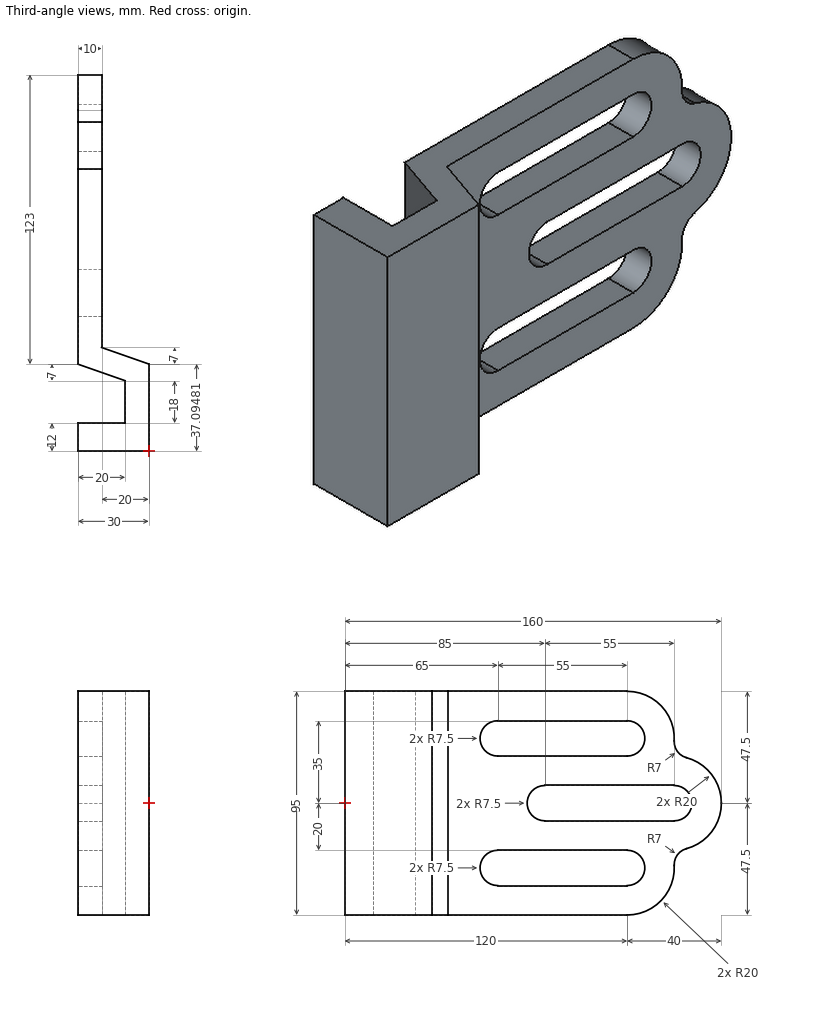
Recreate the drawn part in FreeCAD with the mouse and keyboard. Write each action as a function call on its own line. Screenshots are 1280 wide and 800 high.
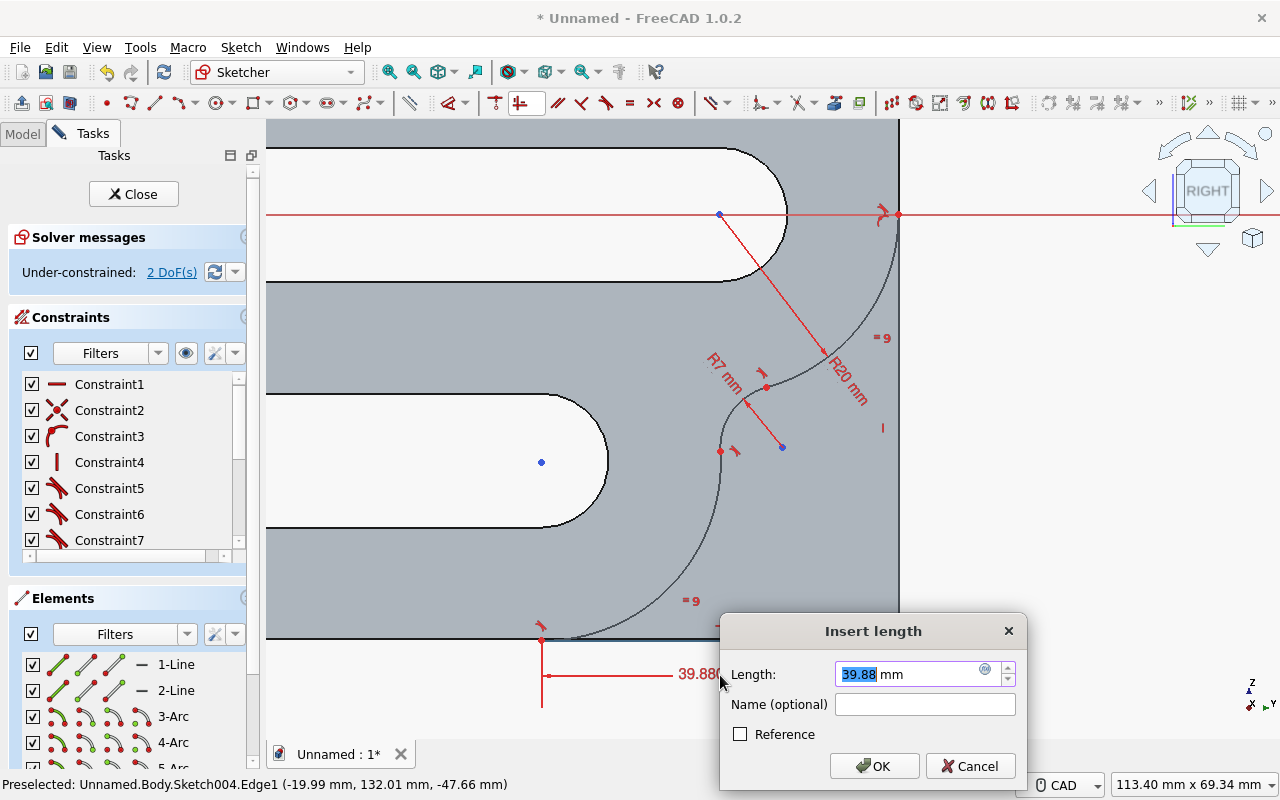
text(40)
key(Return)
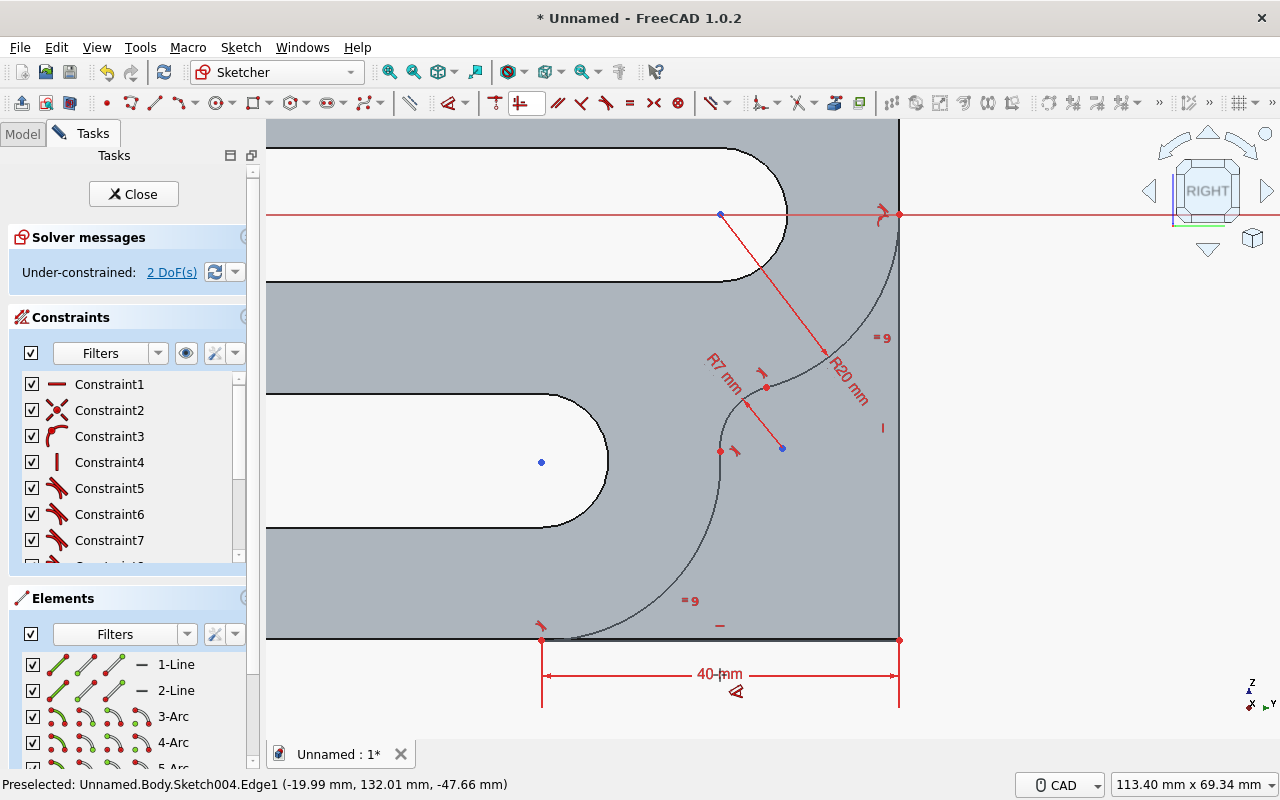
click(899, 513)
click(933, 428)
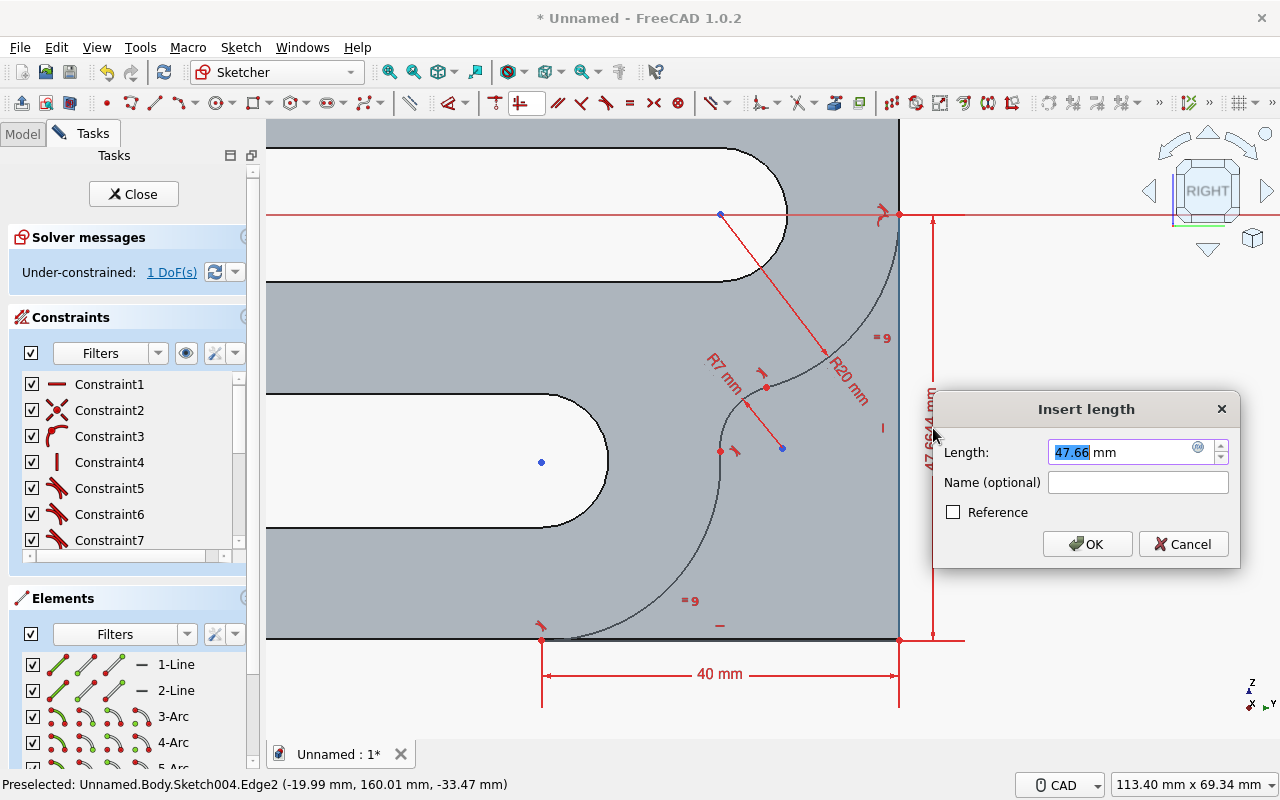
text(47.5)
key(Return)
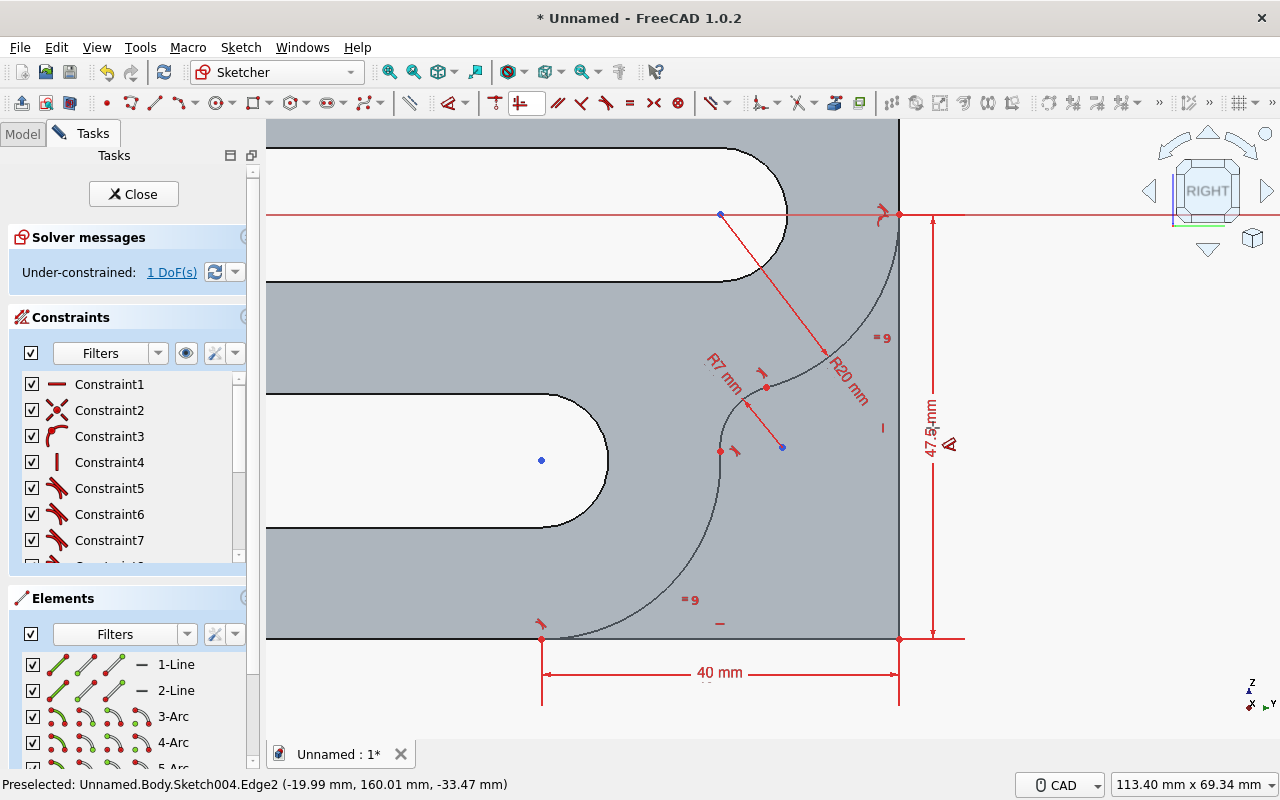
click(542, 639)
click(418, 673)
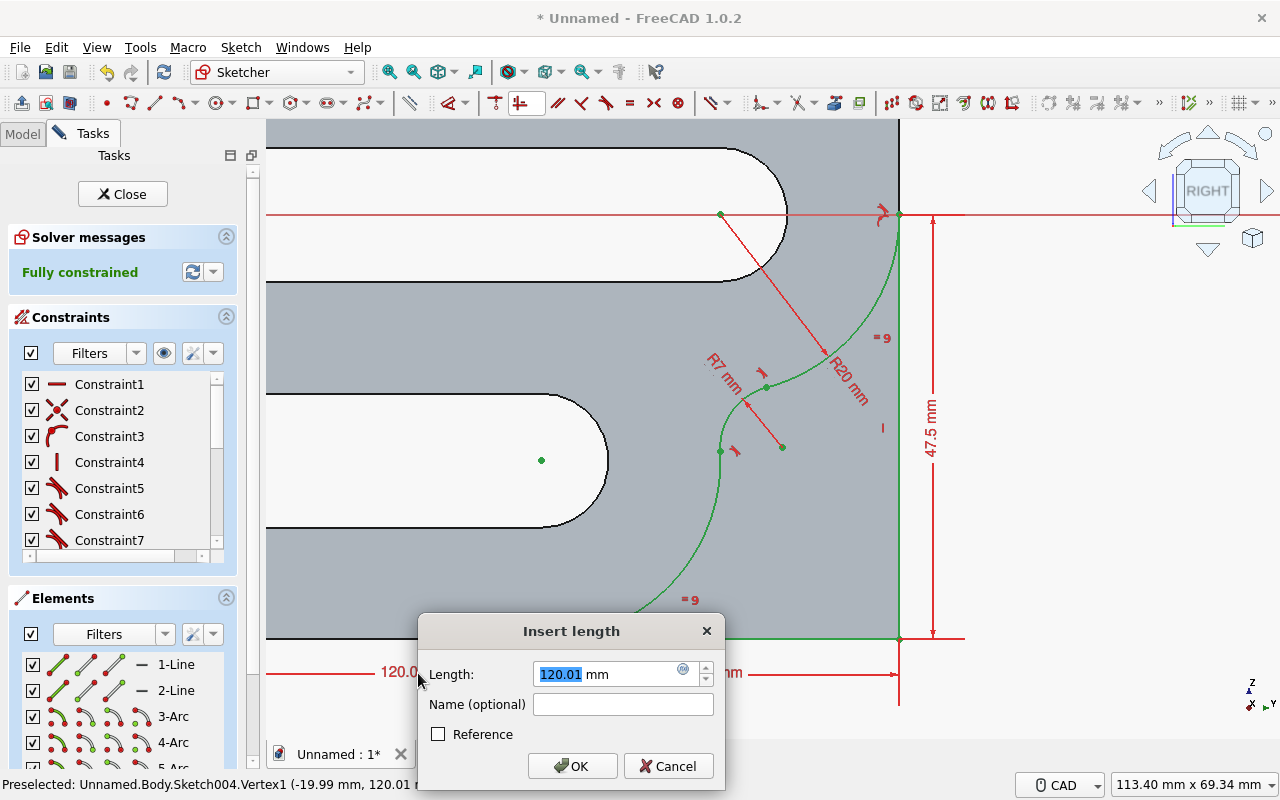
text(120)
key(Return)
key(Escape)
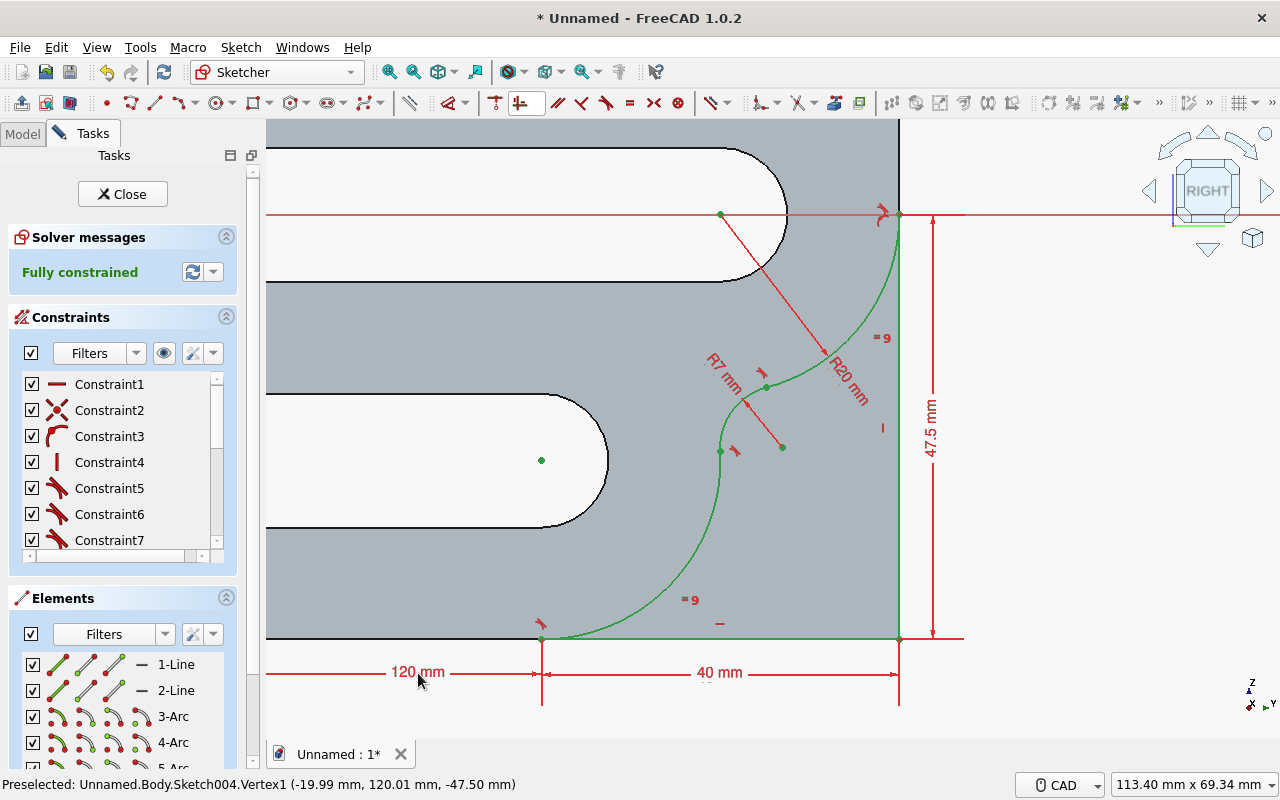
click(123, 194)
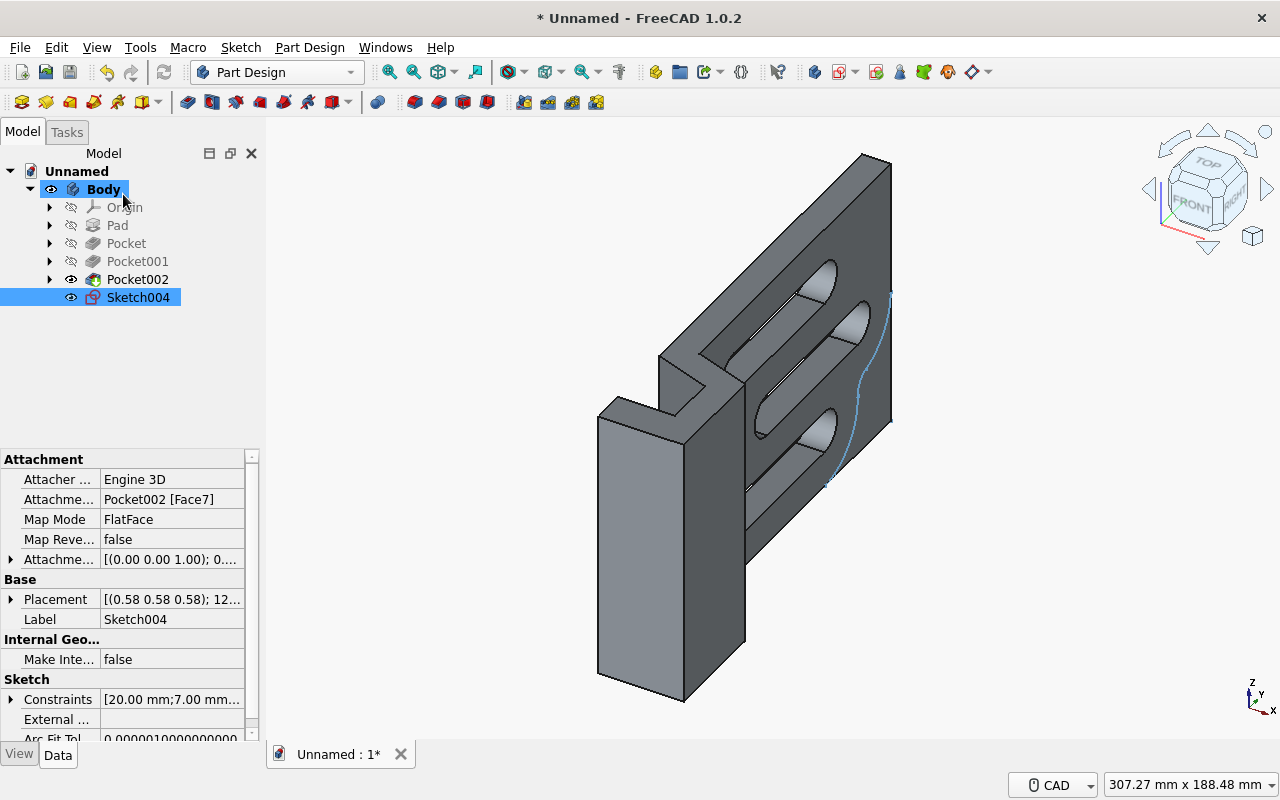
click(188, 102)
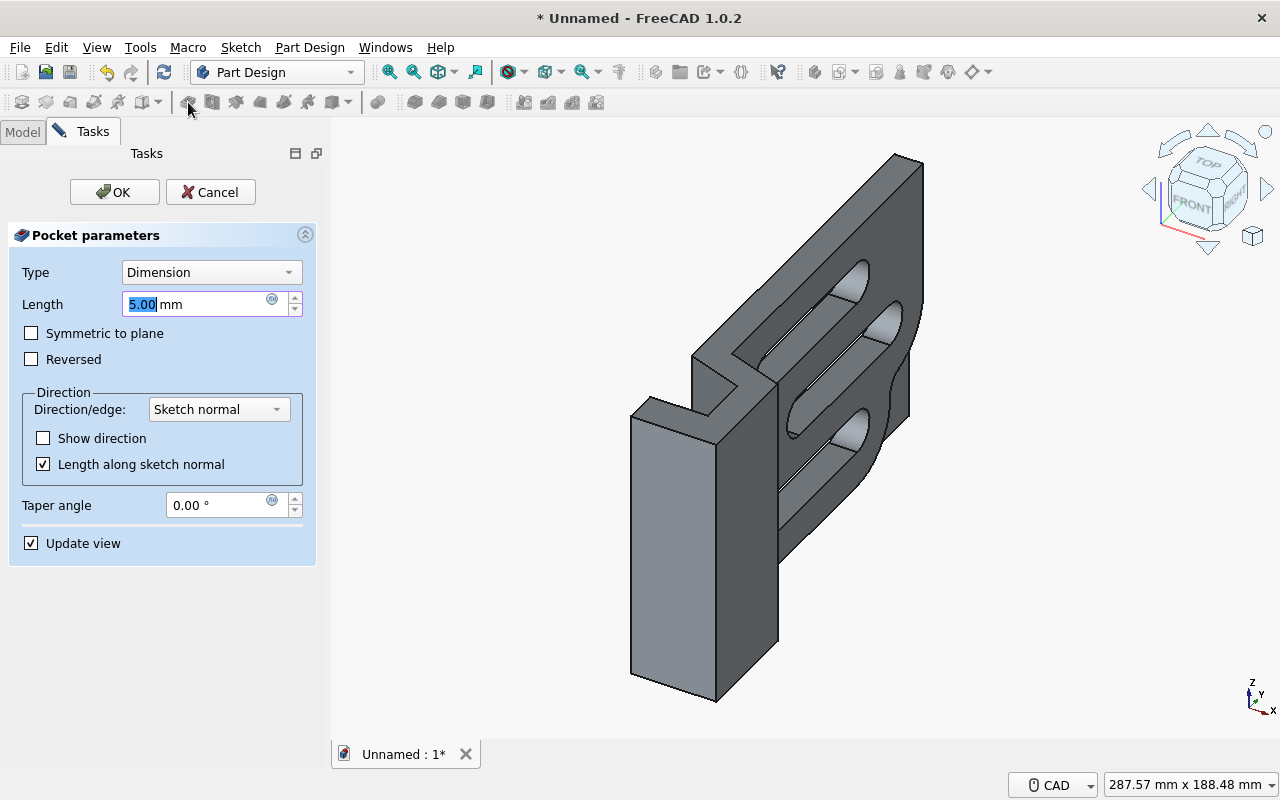
click(212, 272)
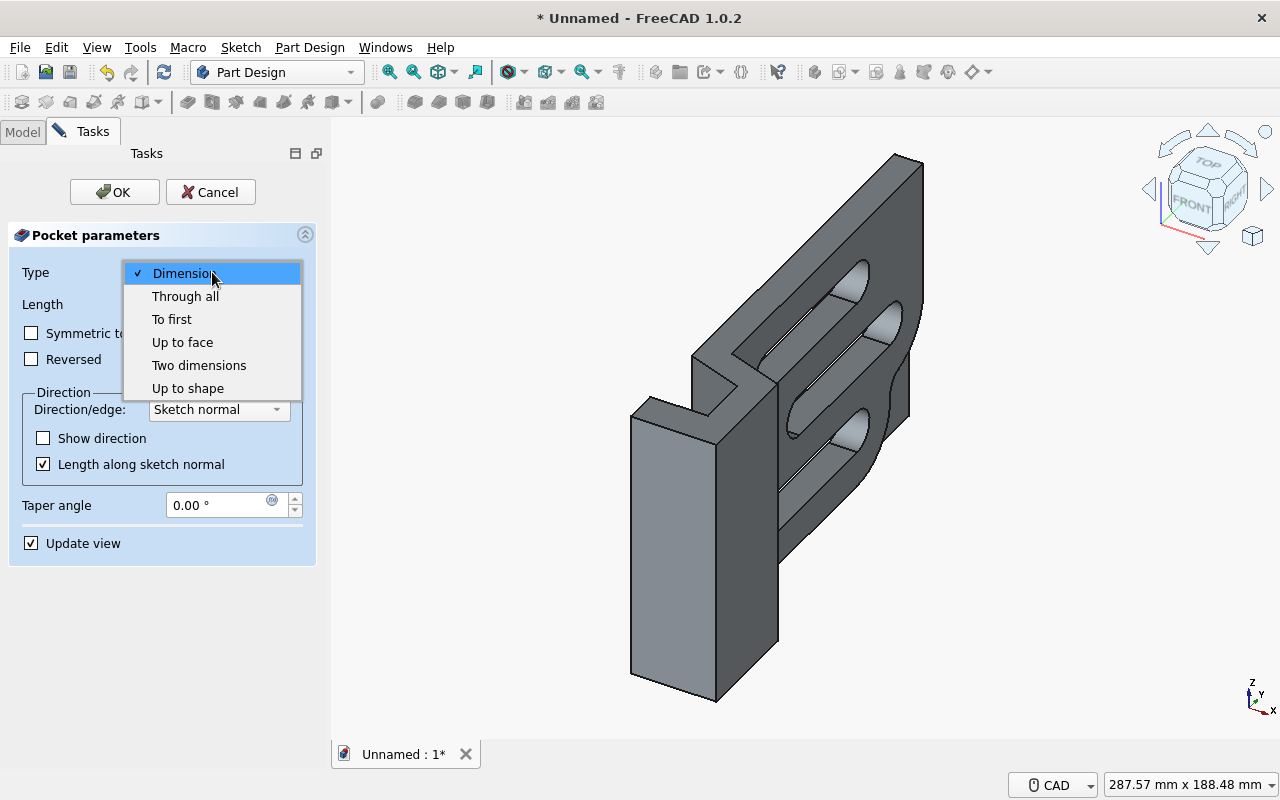
click(212, 320)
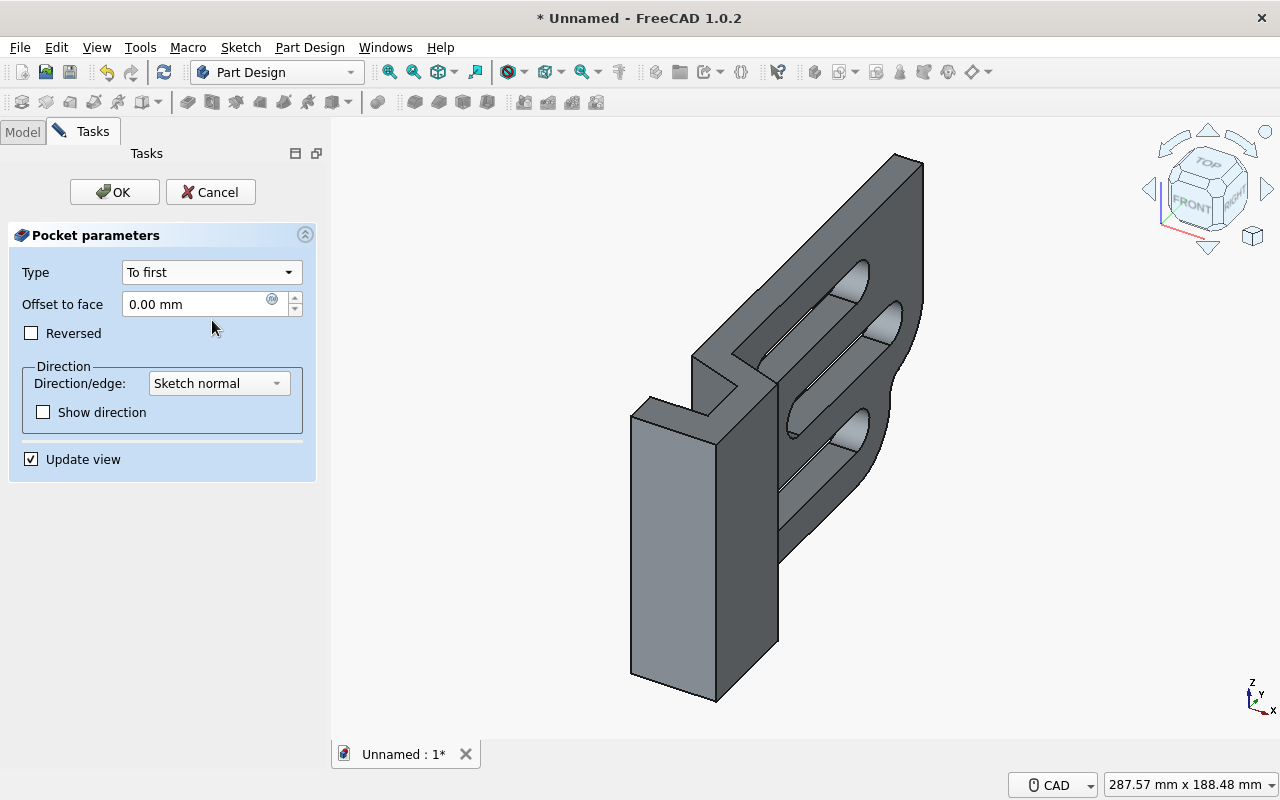
click(115, 192)